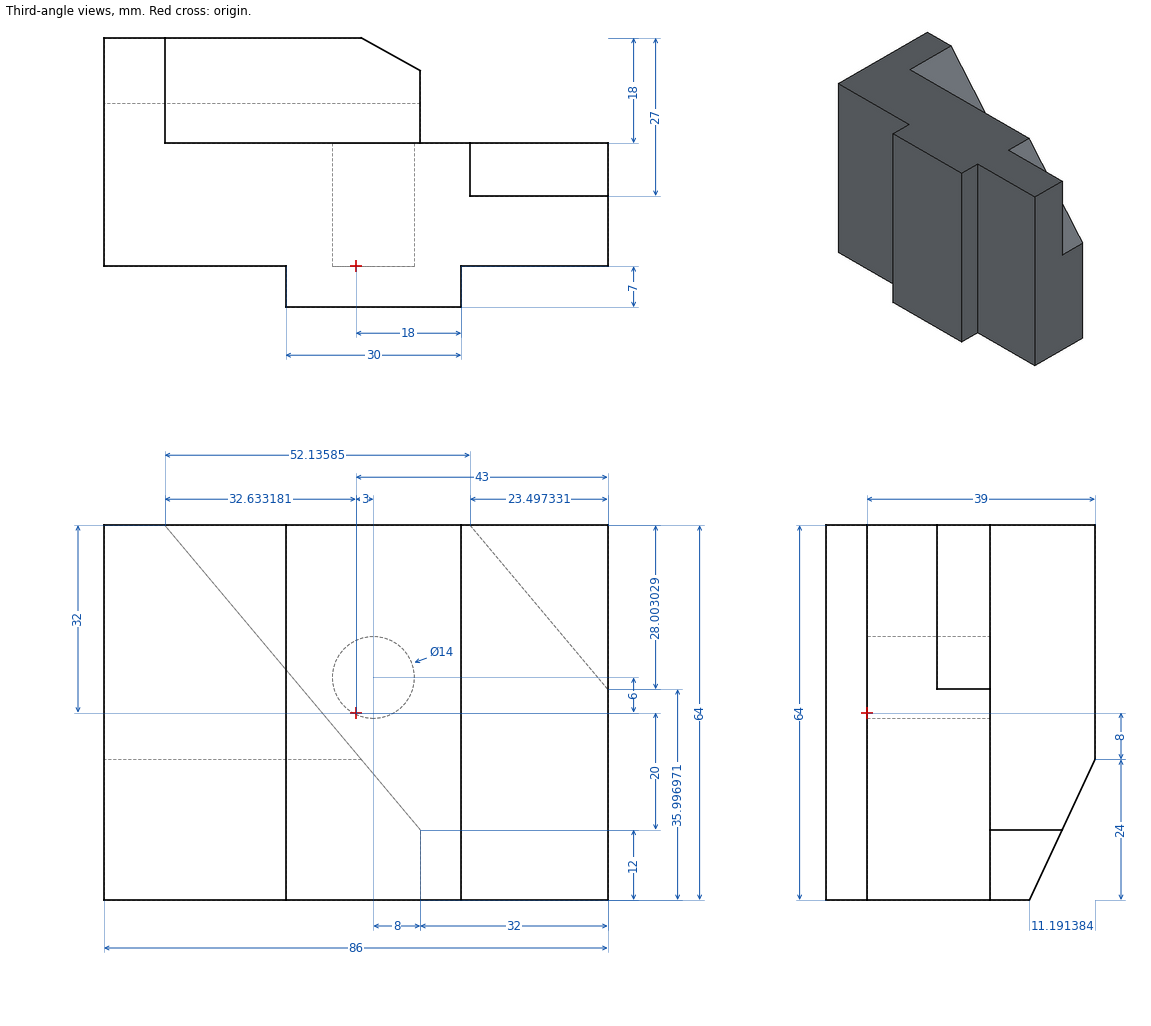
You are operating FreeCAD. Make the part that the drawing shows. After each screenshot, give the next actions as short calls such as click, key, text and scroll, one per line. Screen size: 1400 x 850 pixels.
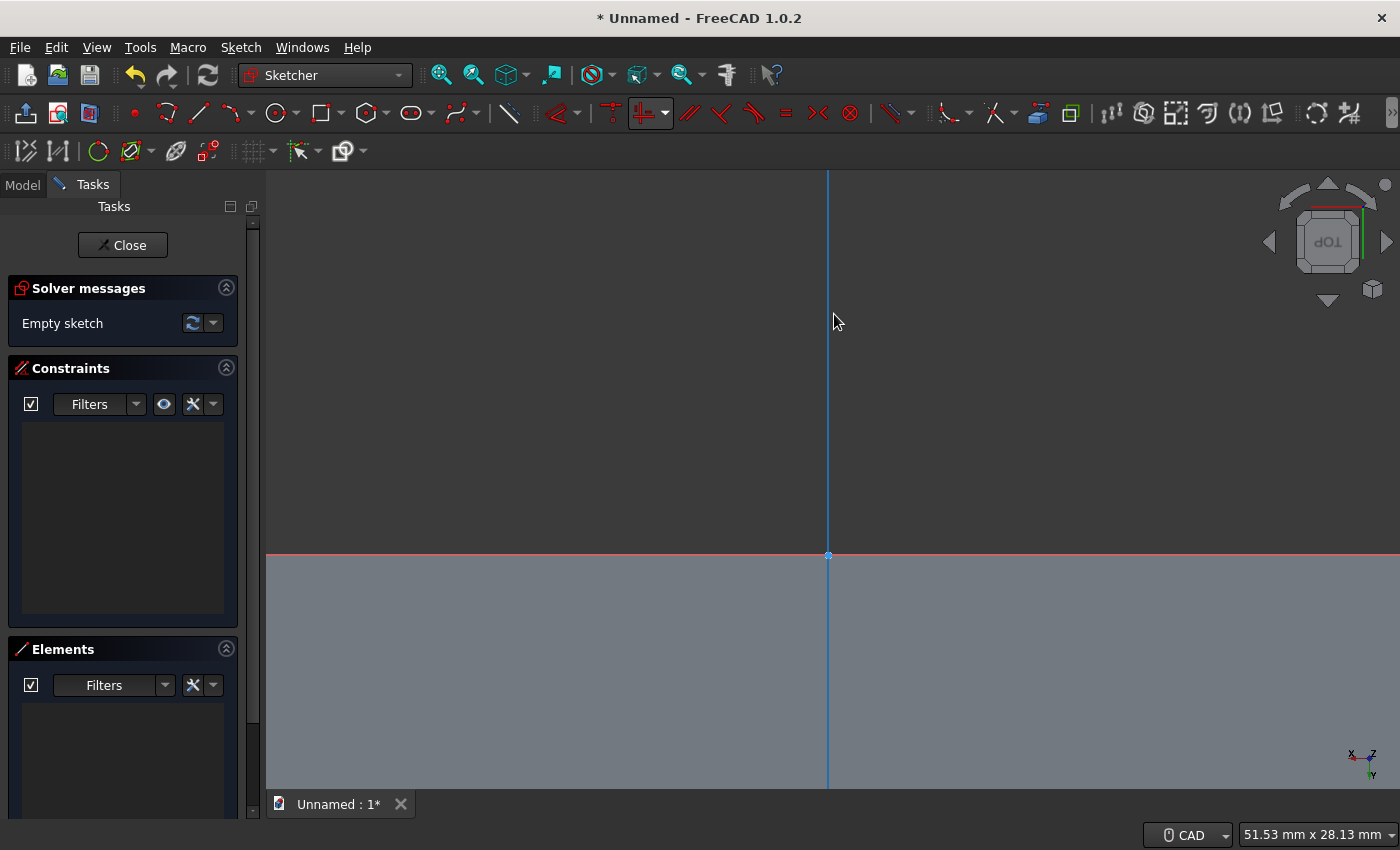
click(322, 114)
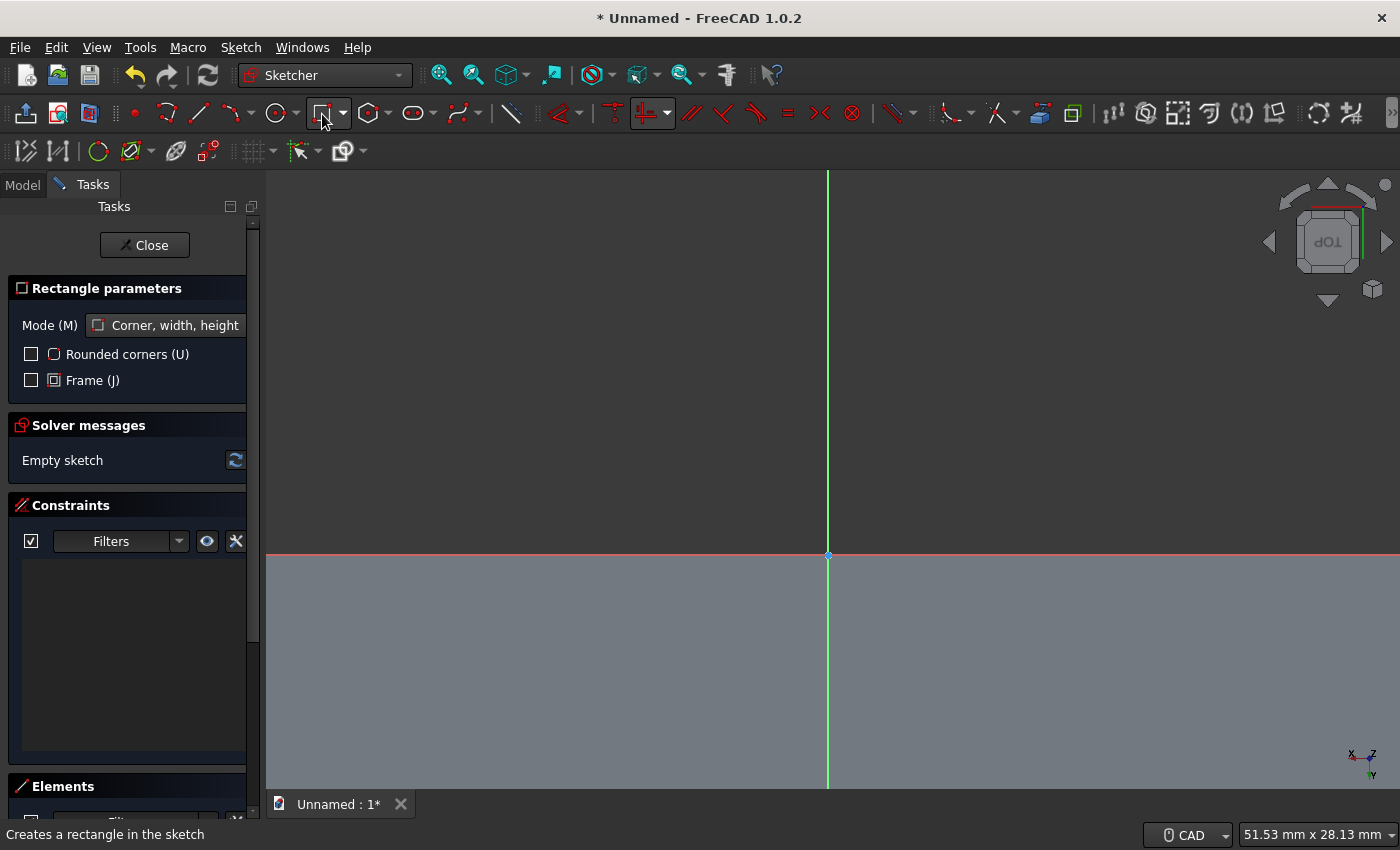
click(432, 401)
click(1092, 555)
key(Escape)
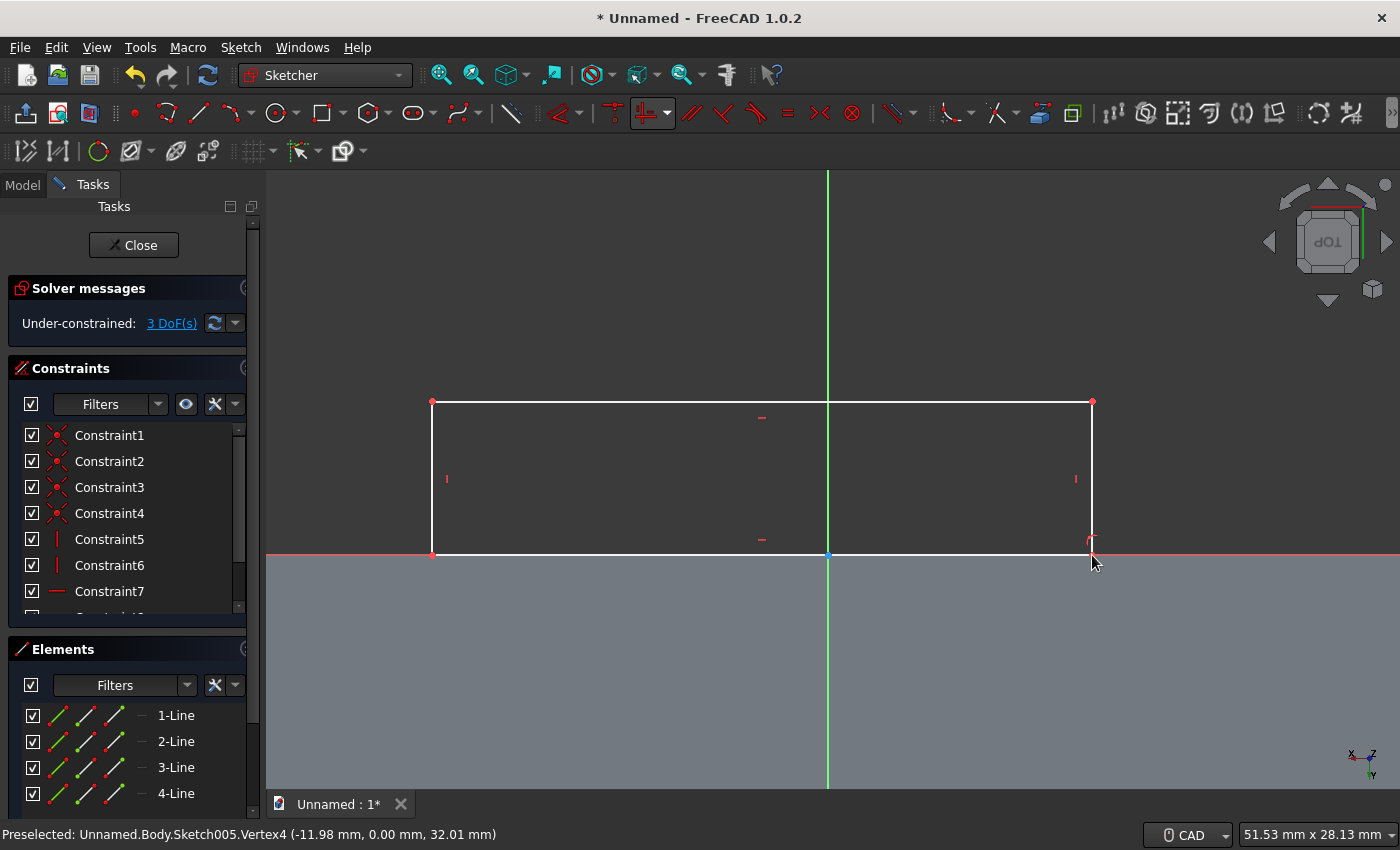
key(d)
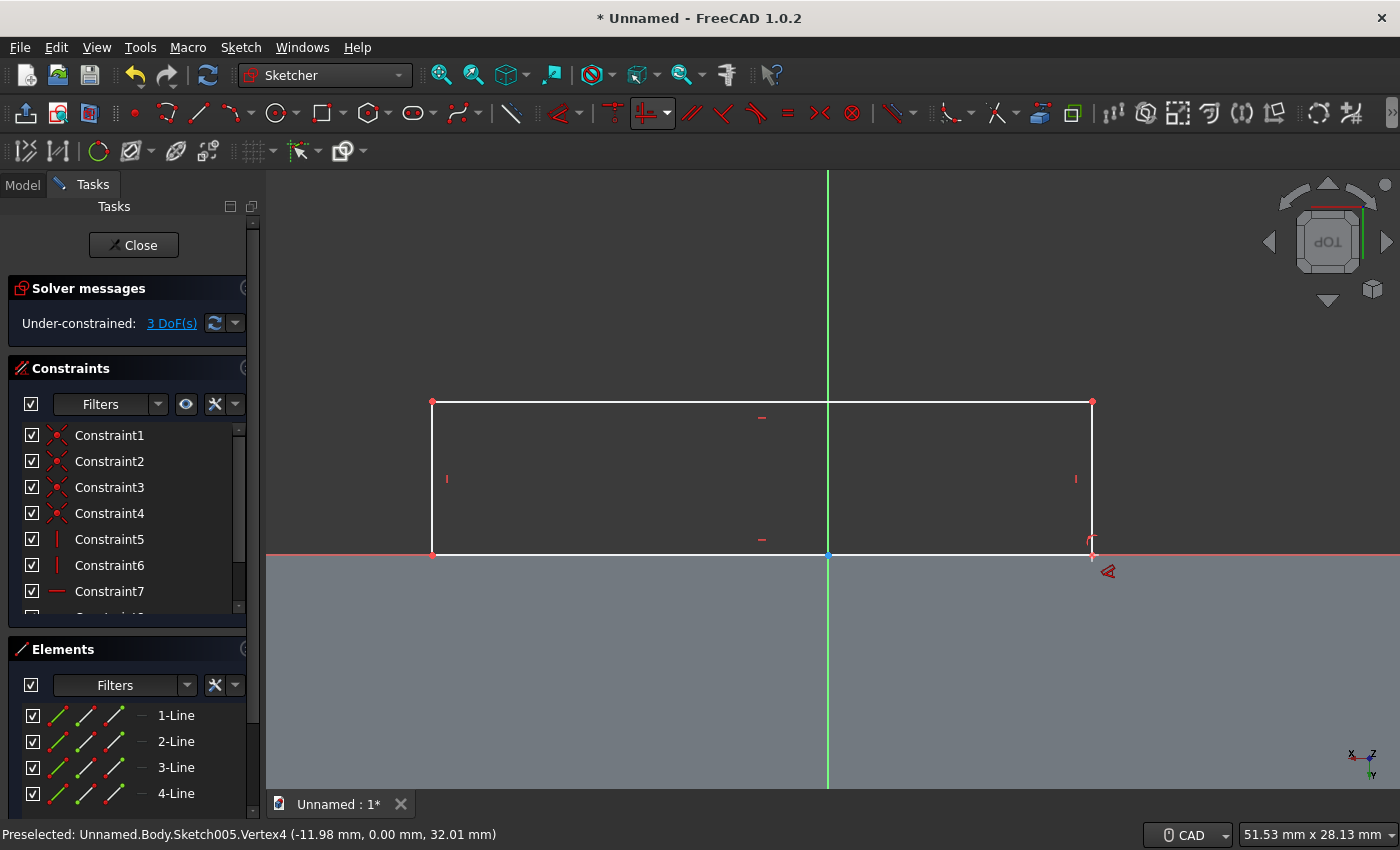
click(432, 448)
click(398, 479)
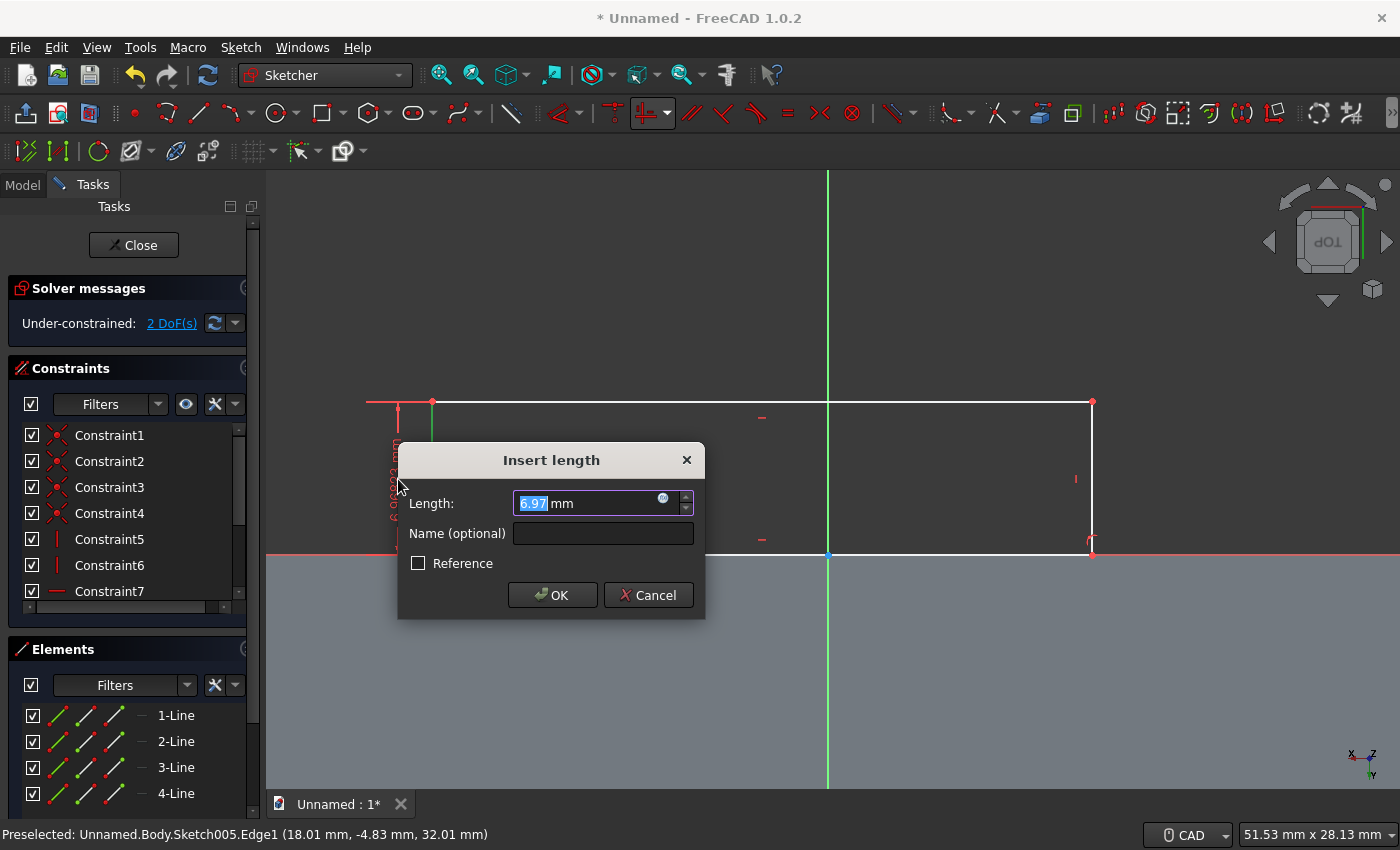
text(7)
key(Return)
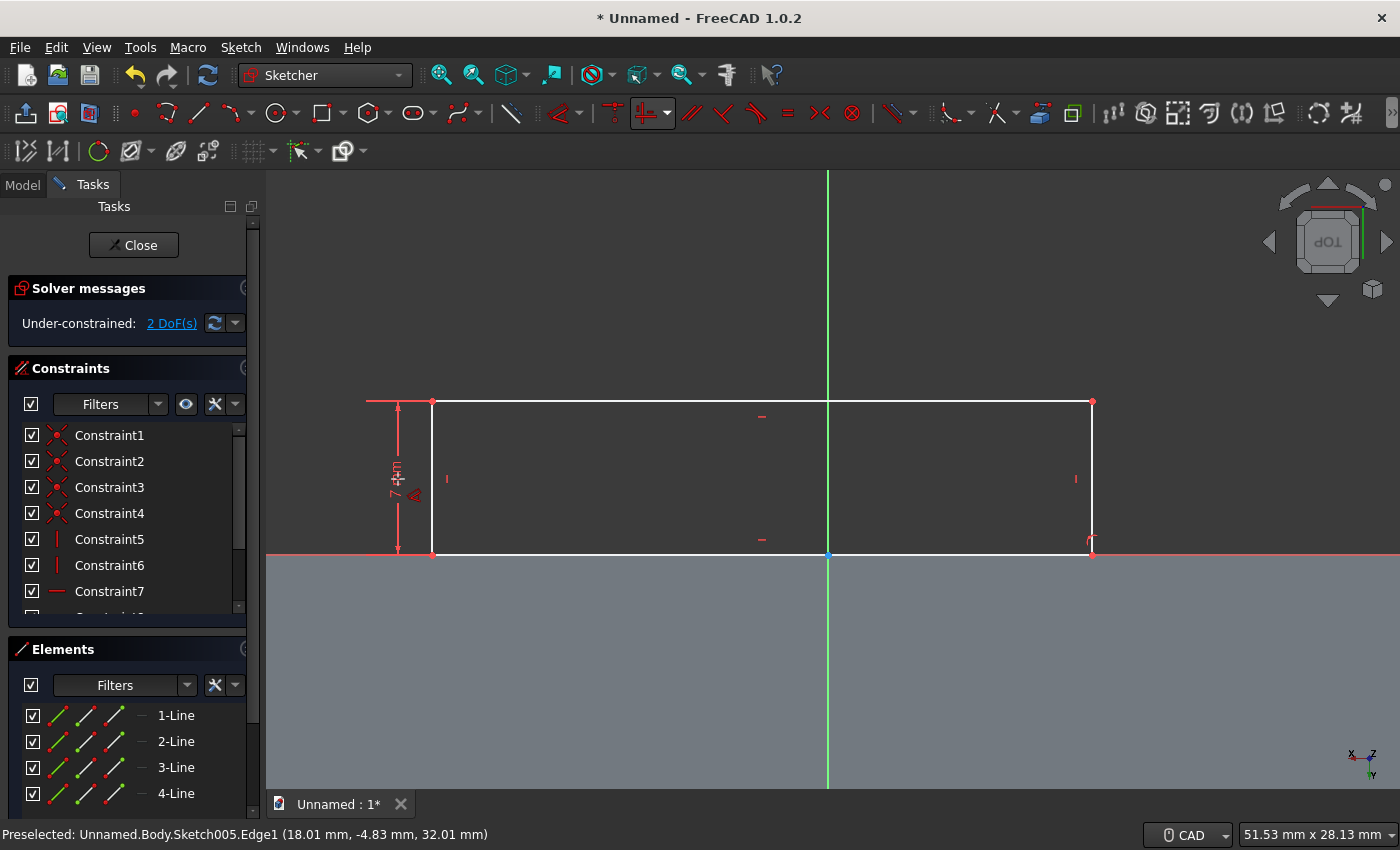
click(630, 555)
click(762, 589)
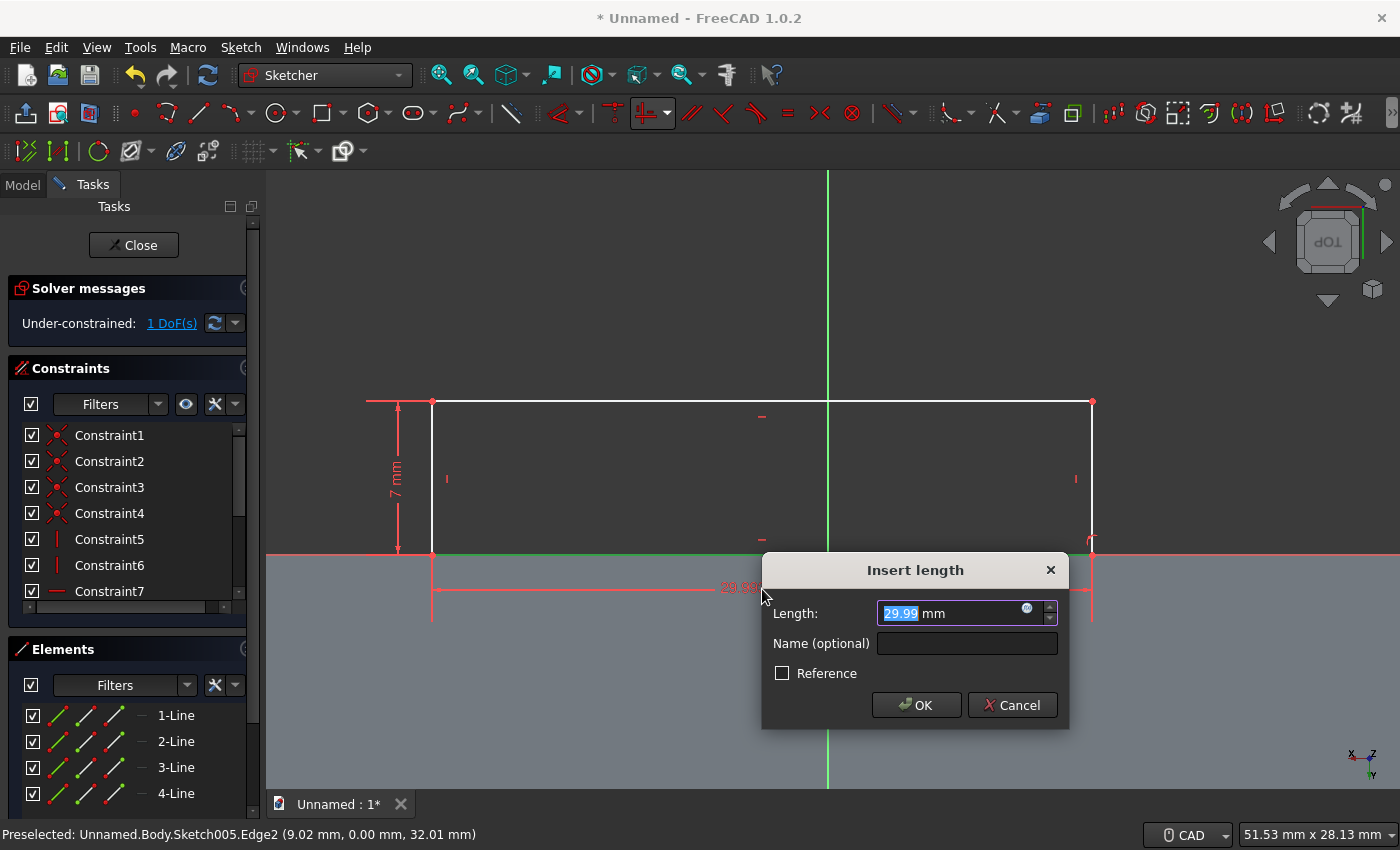
text(30)
key(Return)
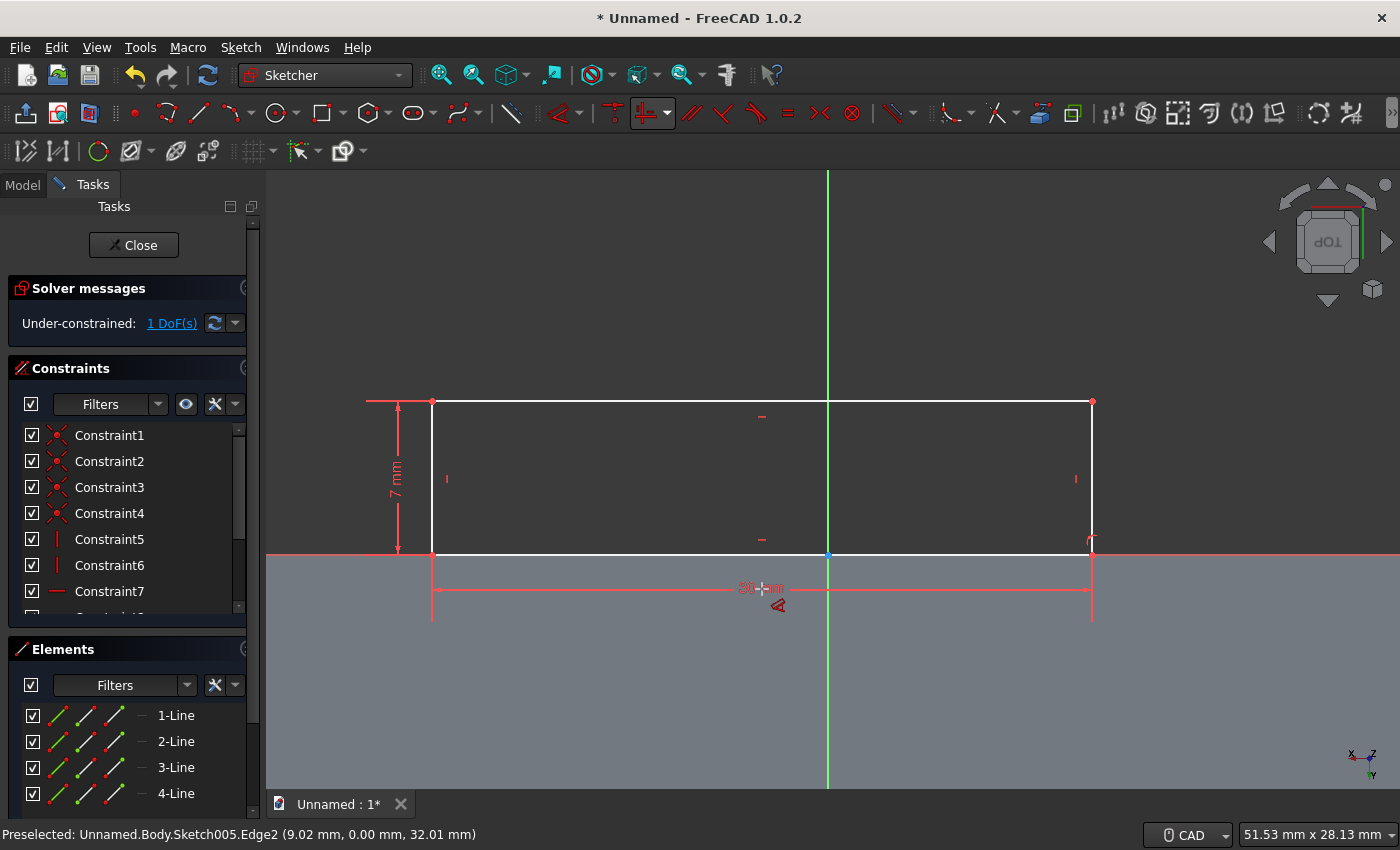
click(432, 401)
click(630, 589)